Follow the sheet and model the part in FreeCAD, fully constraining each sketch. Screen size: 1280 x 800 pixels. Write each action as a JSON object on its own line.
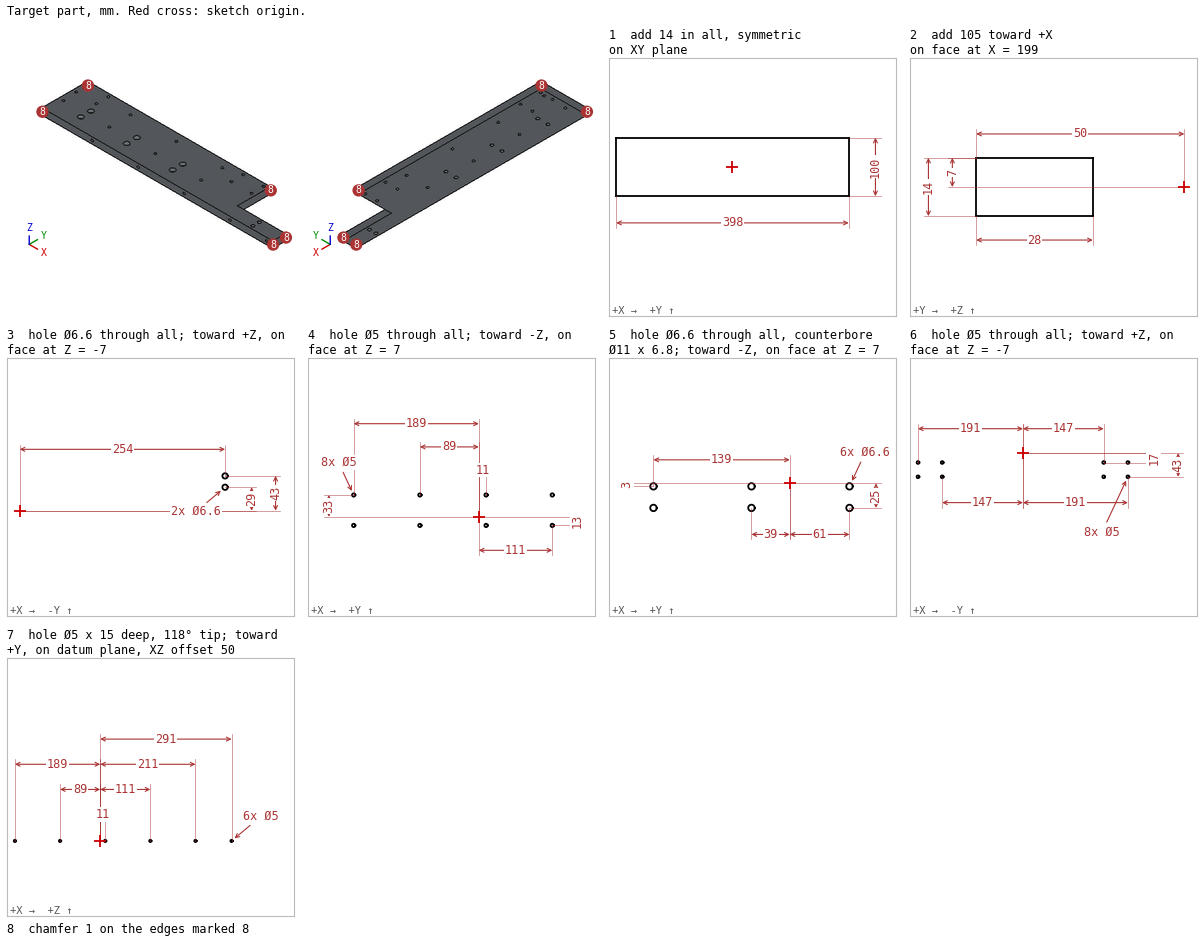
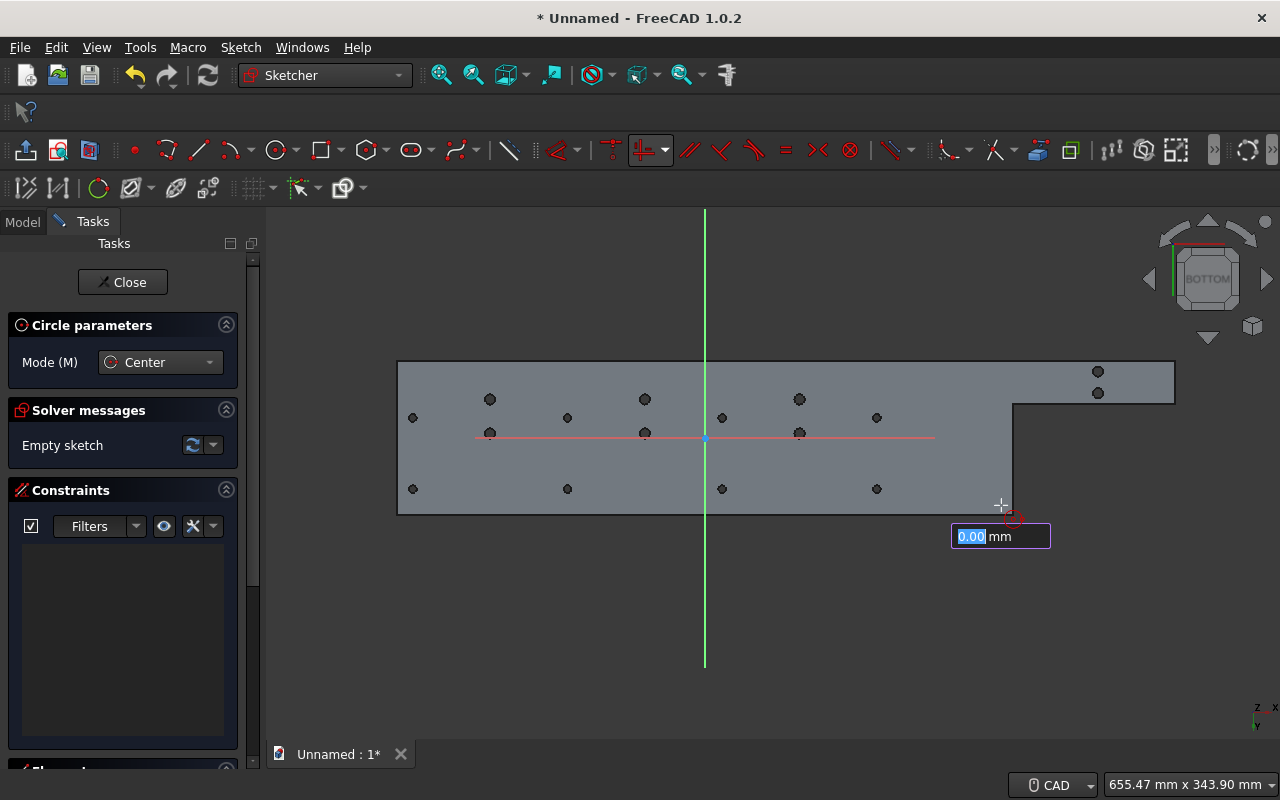
{"action": "scroll", "coordinate": [1003, 502], "scroll_direction": "up", "scroll_amount": 8}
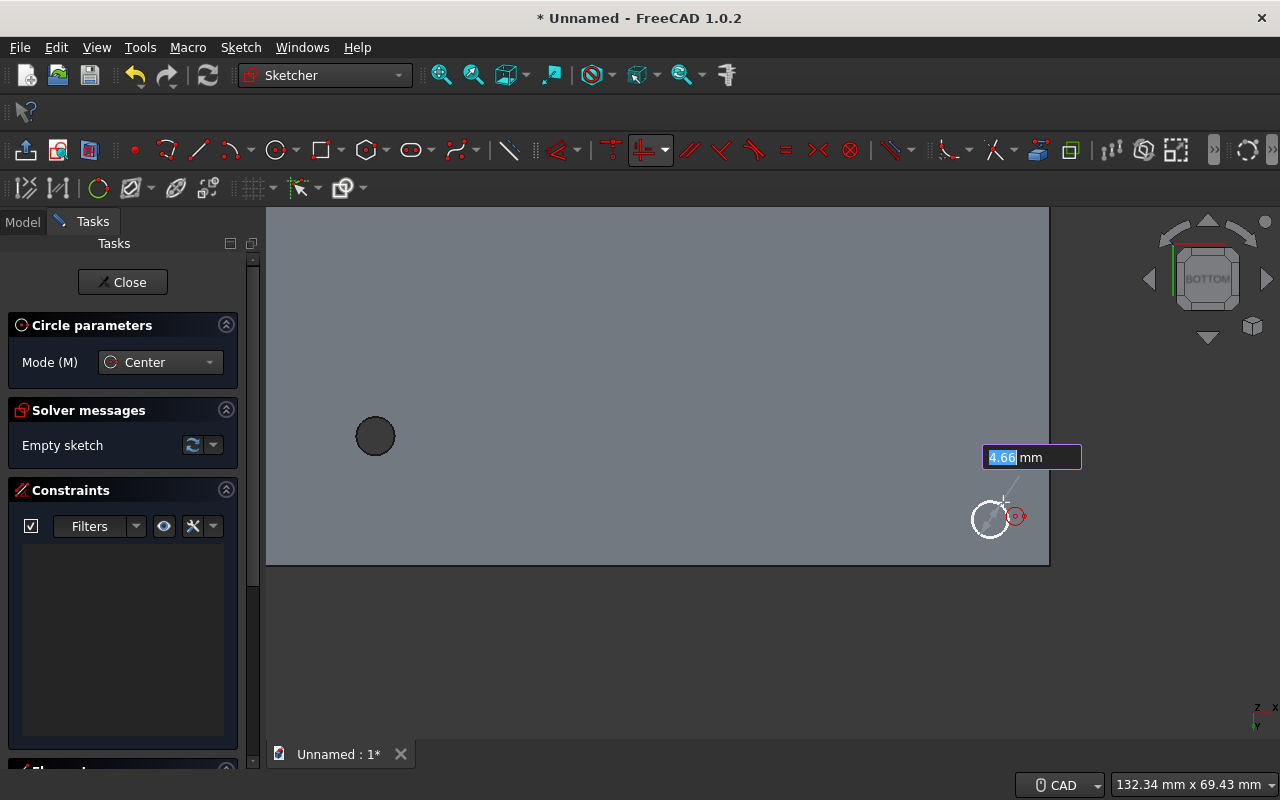
{"action": "left_click", "coordinate": [1002, 499]}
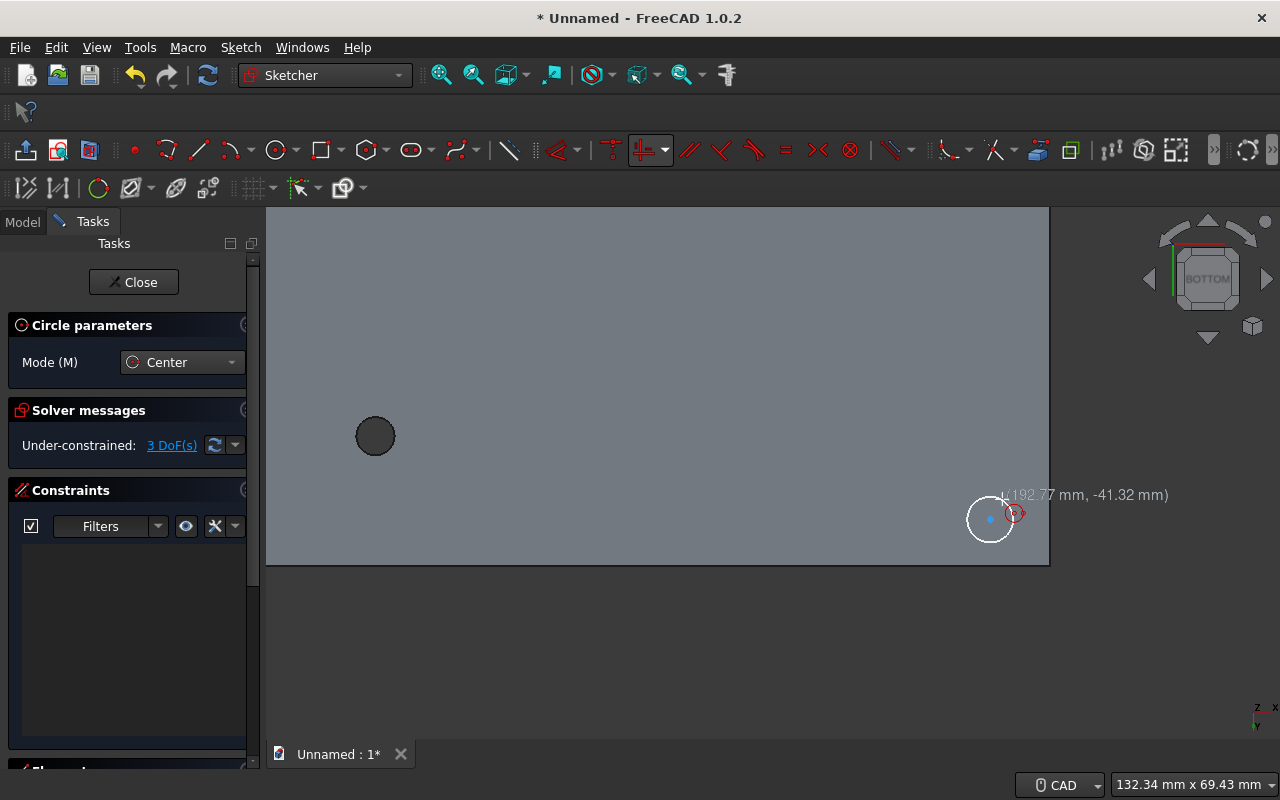
{"action": "scroll", "coordinate": [1003, 502], "scroll_direction": "down", "scroll_amount": 8}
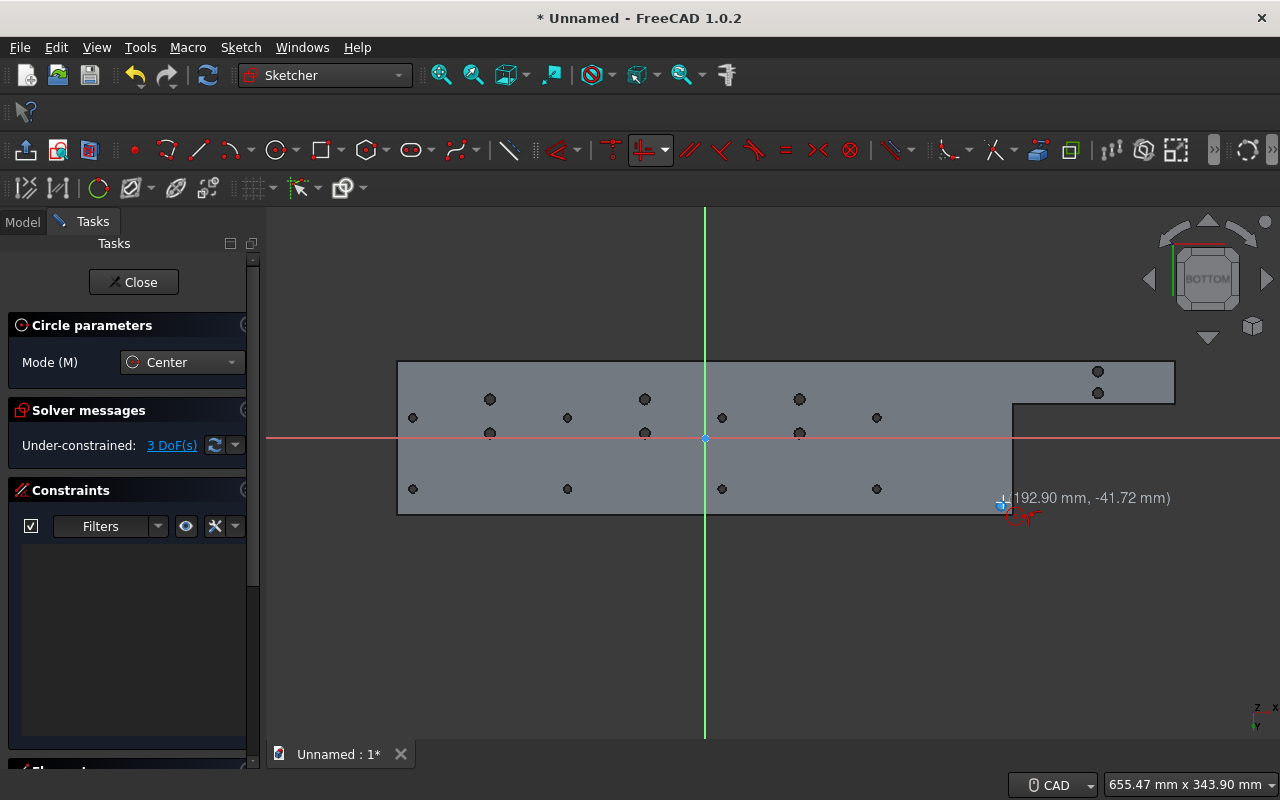
{"action": "left_click", "coordinate": [933, 464]}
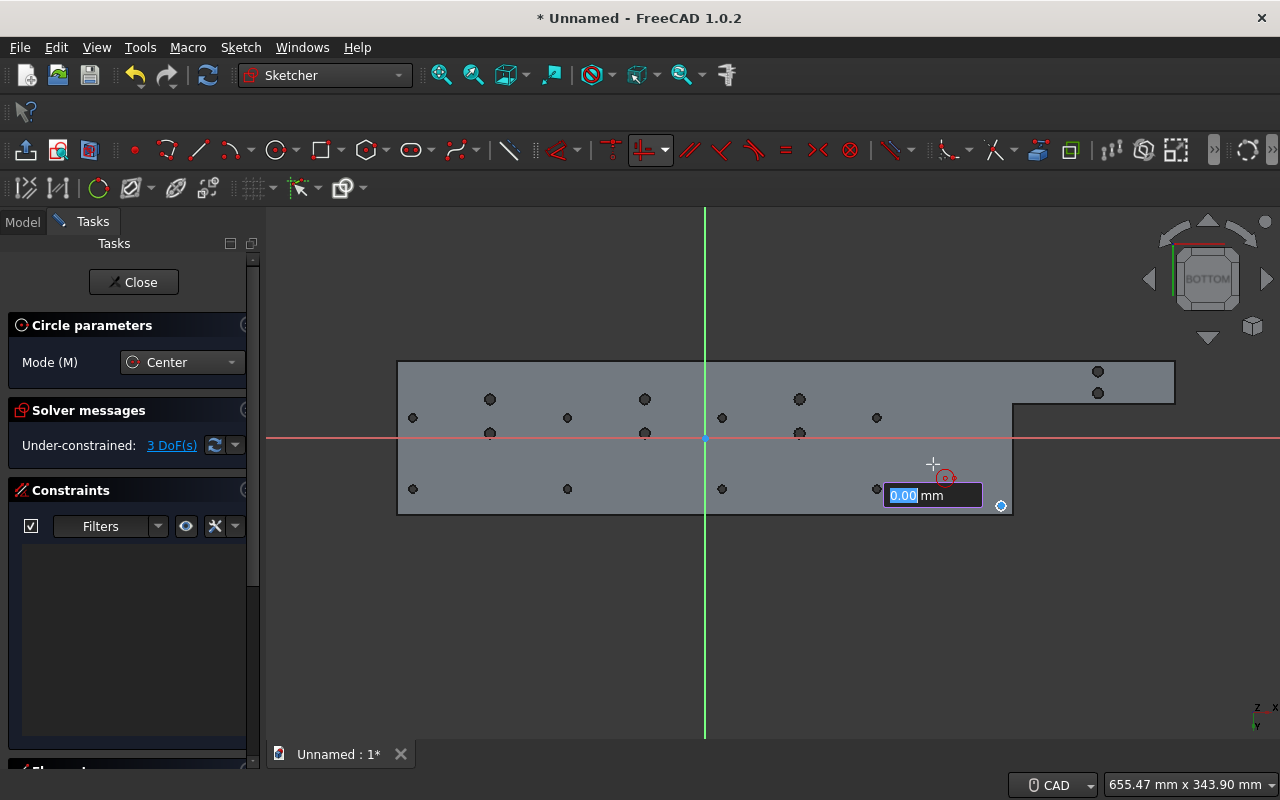
{"action": "scroll", "coordinate": [935, 462], "scroll_direction": "up", "scroll_amount": 8}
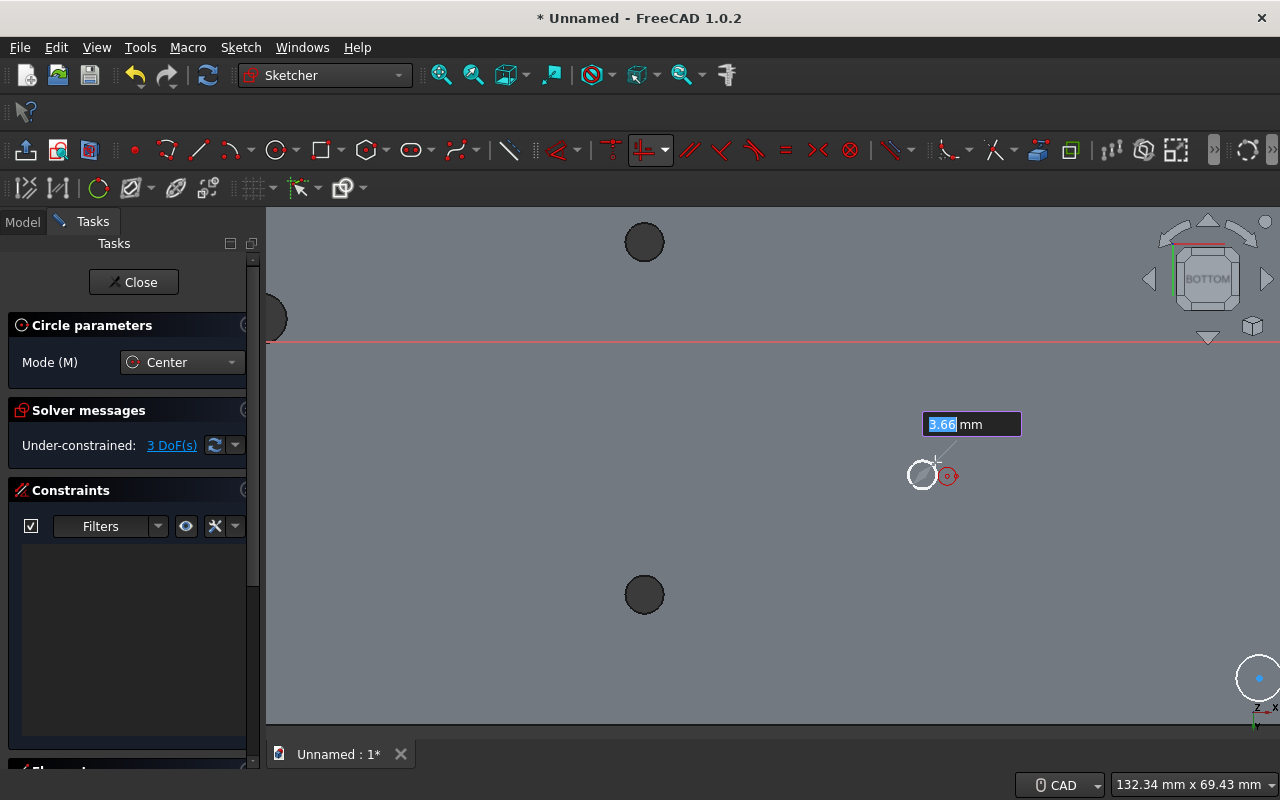
{"action": "left_click", "coordinate": [934, 458]}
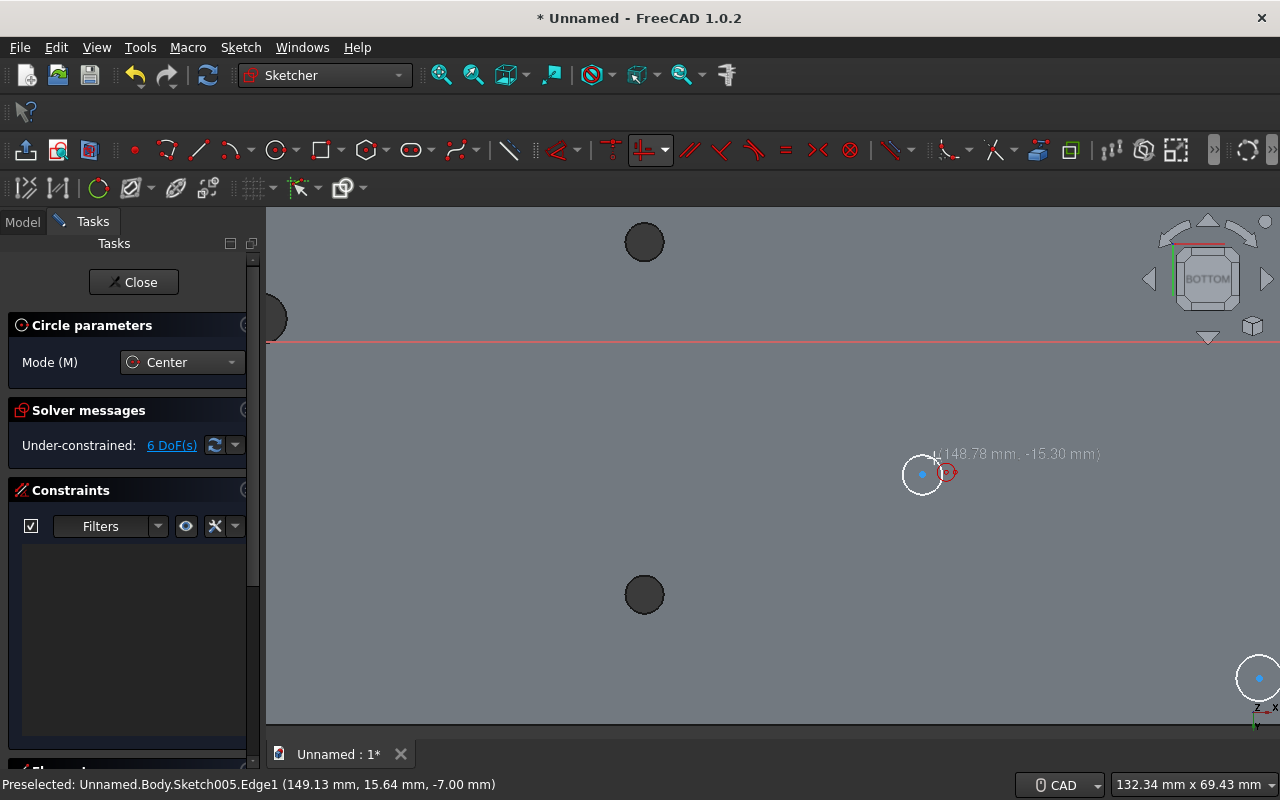
{"action": "scroll", "coordinate": [935, 462], "scroll_direction": "down", "scroll_amount": 8}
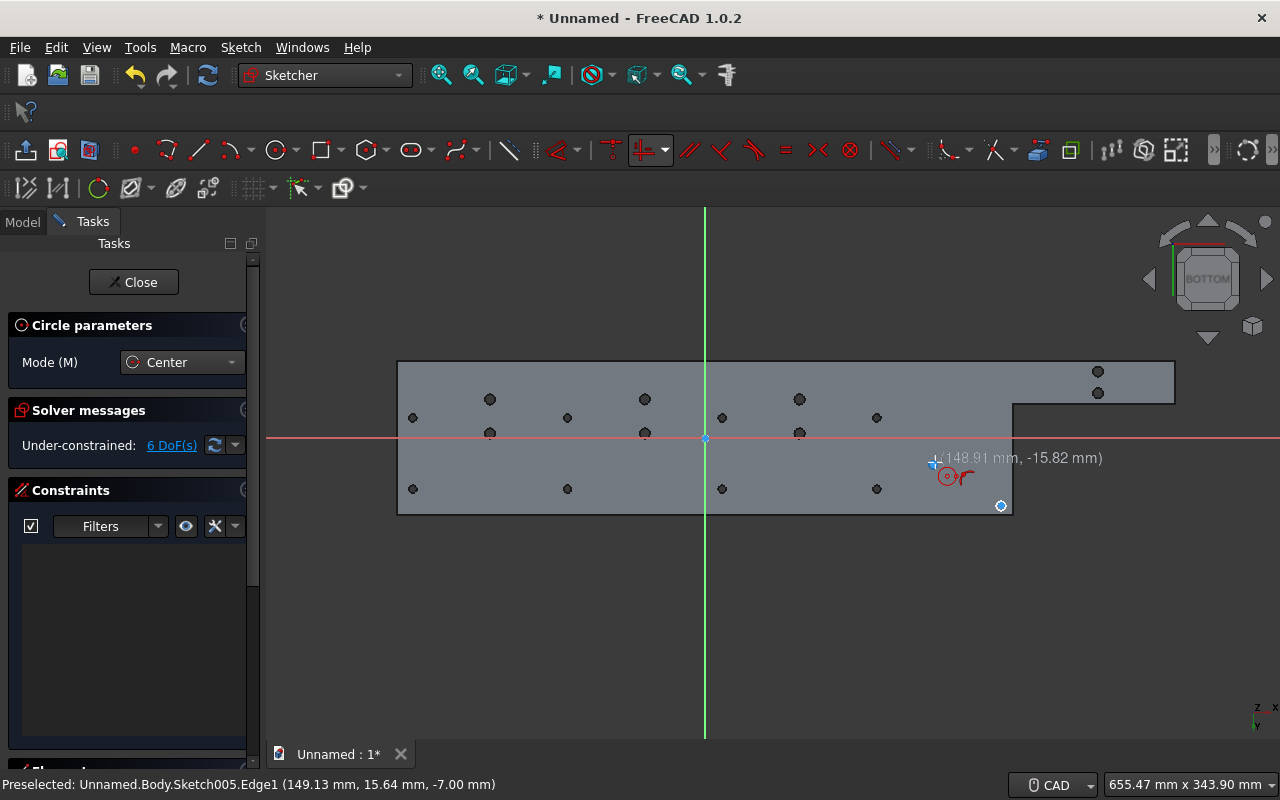
{"action": "scroll", "coordinate": [1001, 464], "scroll_direction": "up", "scroll_amount": 9}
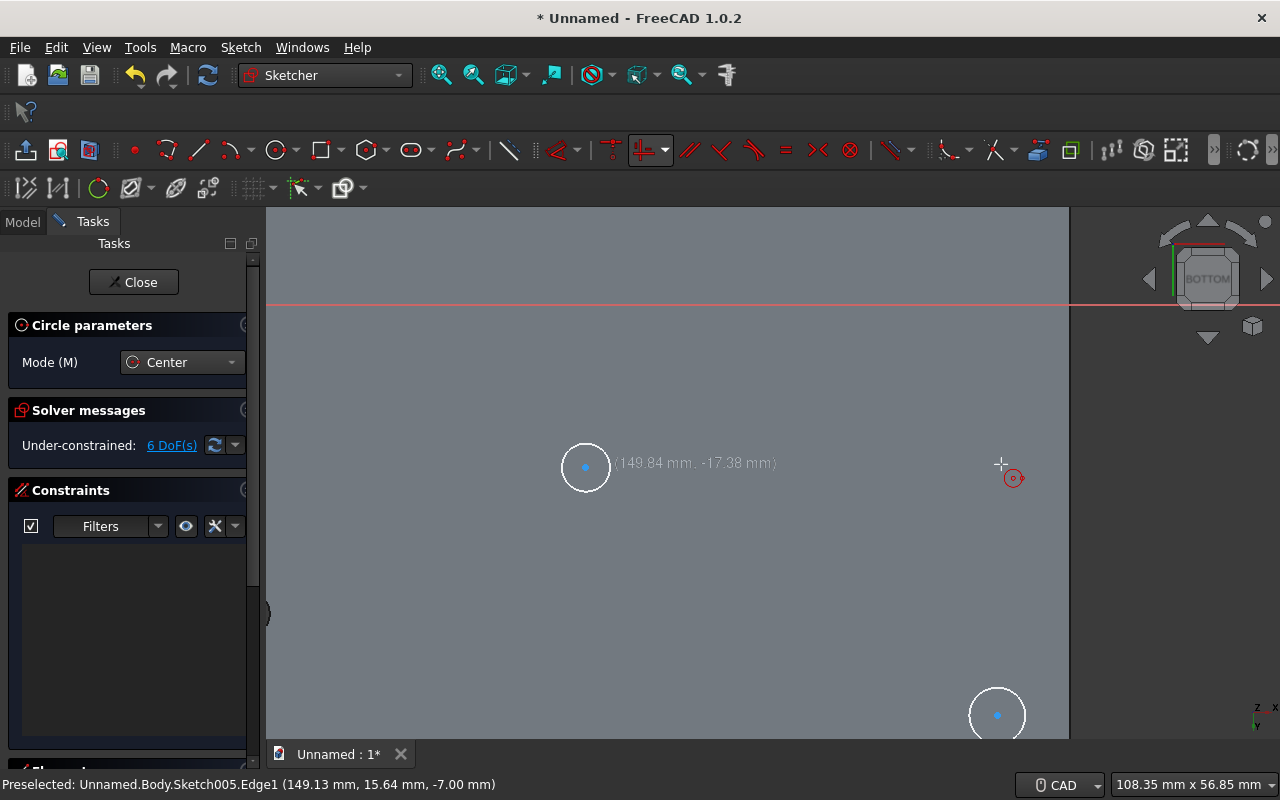
{"action": "scroll", "coordinate": [1001, 464], "scroll_direction": "down", "scroll_amount": 9}